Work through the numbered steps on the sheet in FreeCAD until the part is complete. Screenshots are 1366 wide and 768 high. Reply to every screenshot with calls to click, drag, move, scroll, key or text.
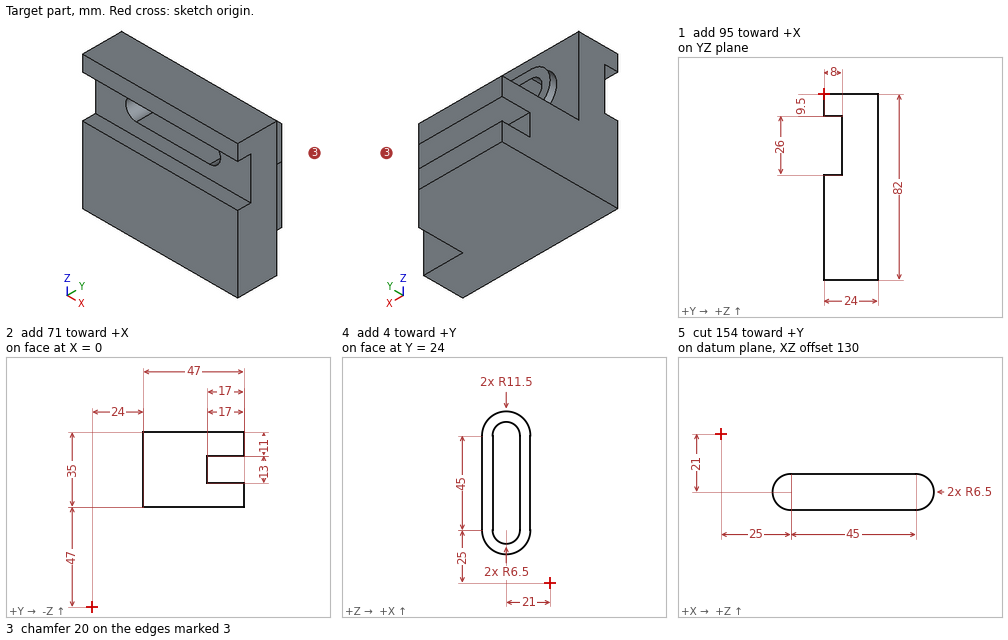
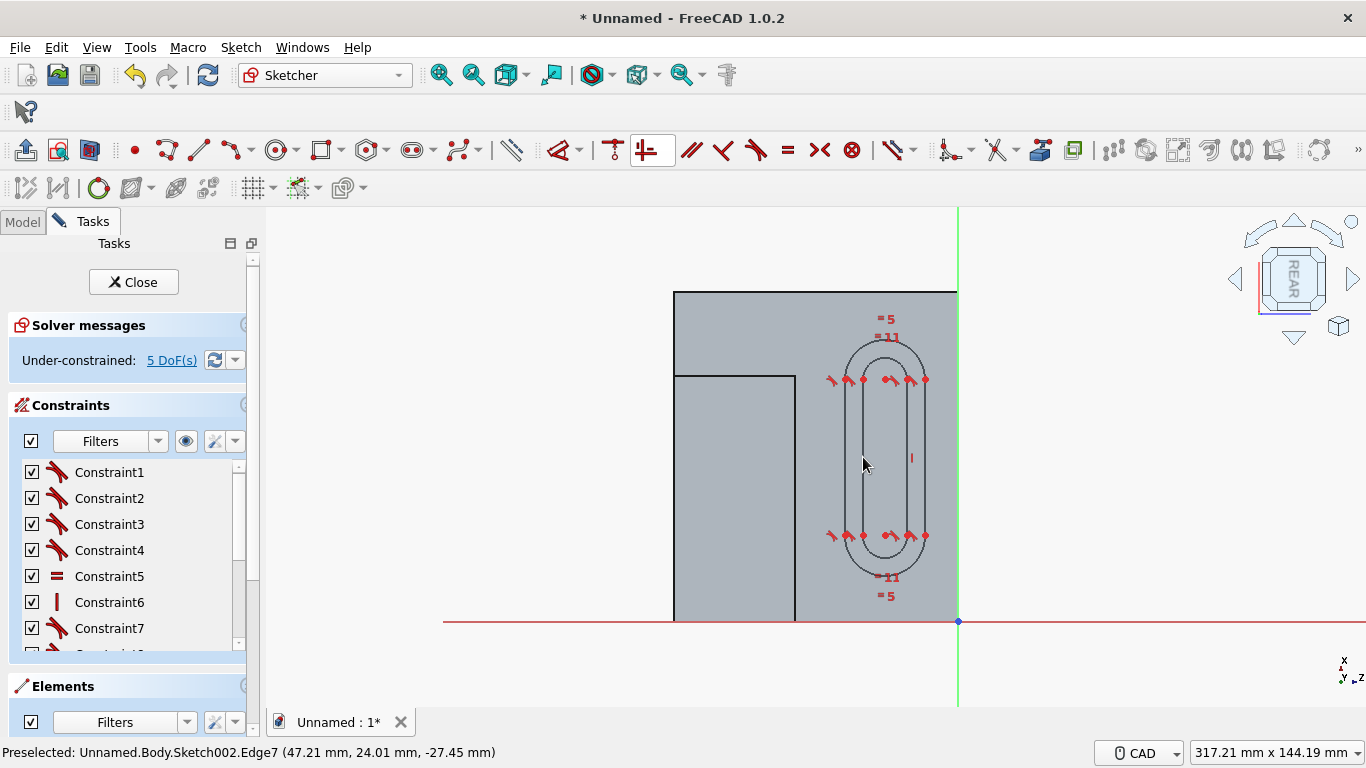
click(558, 150)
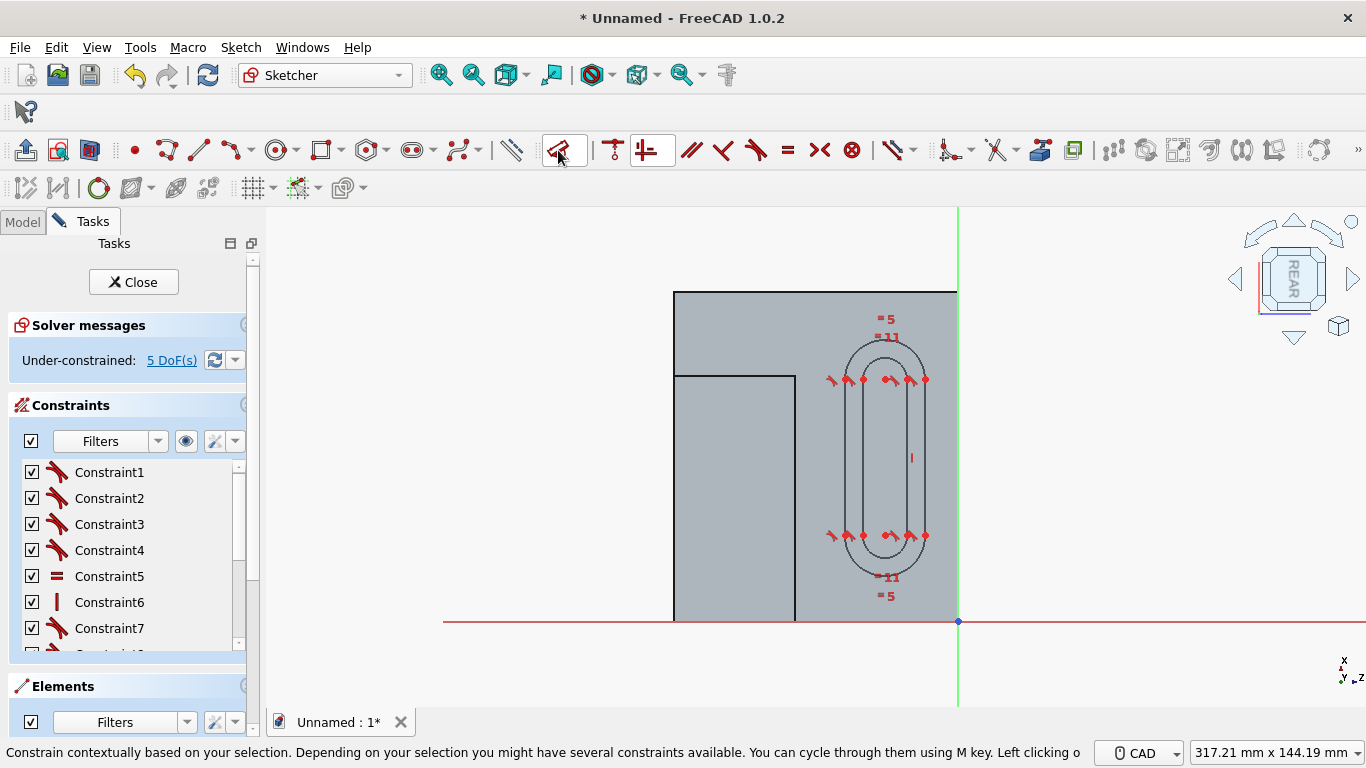
click(861, 568)
click(842, 594)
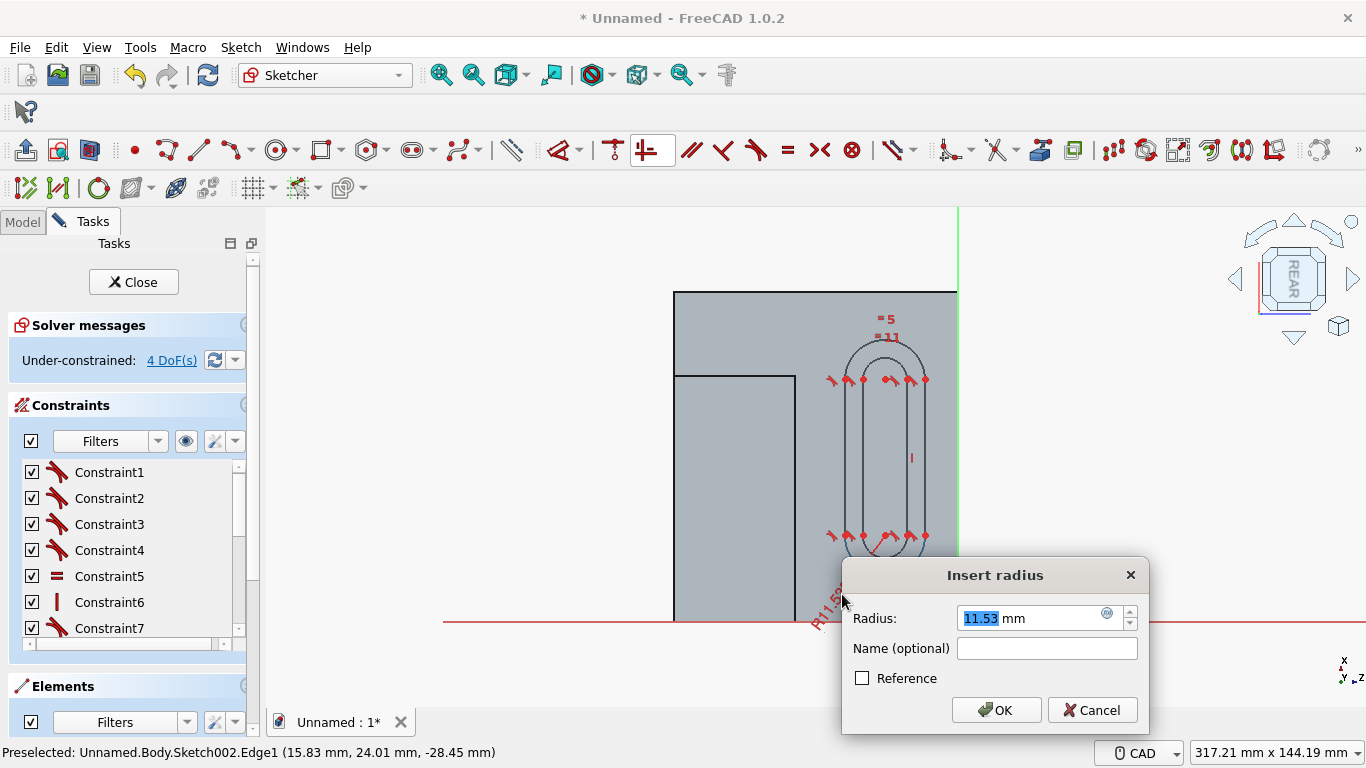
text(11.5)
key(Return)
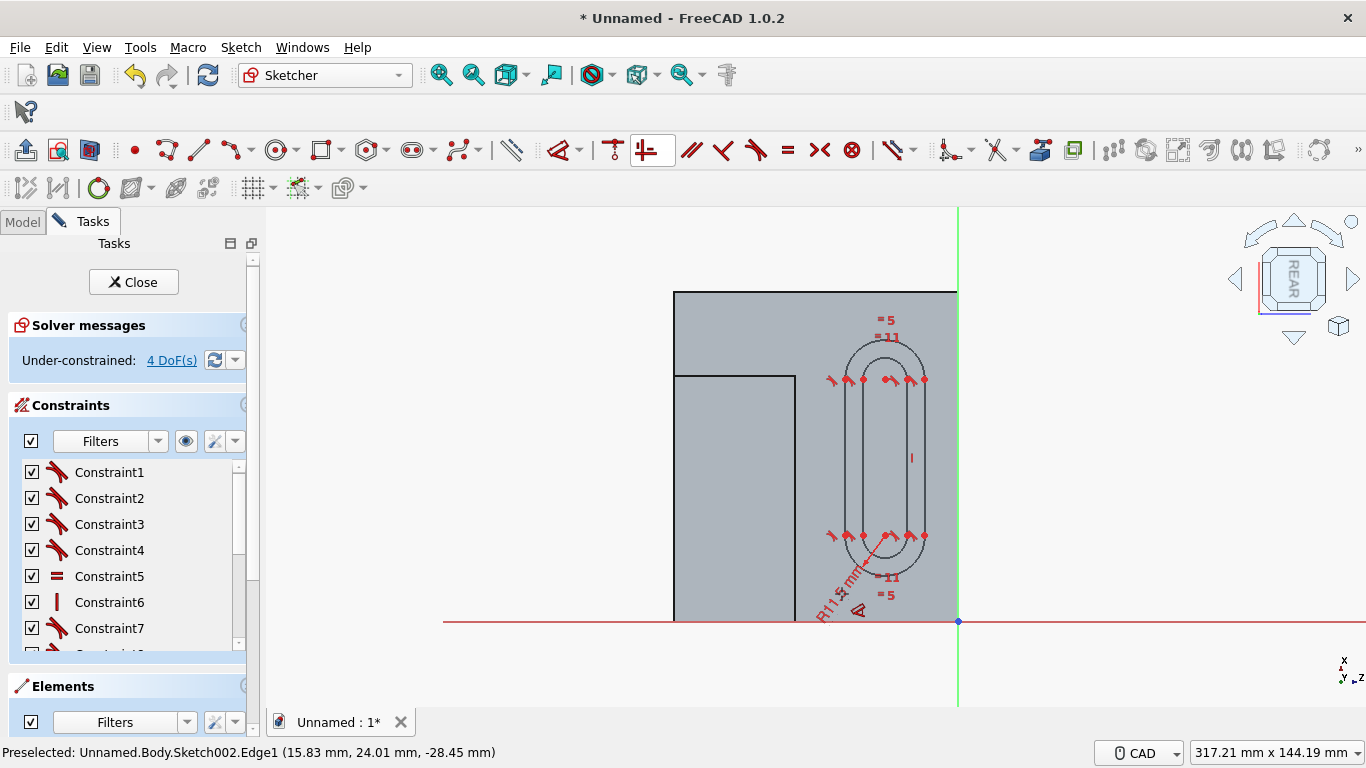
scroll(872, 554, up, 3)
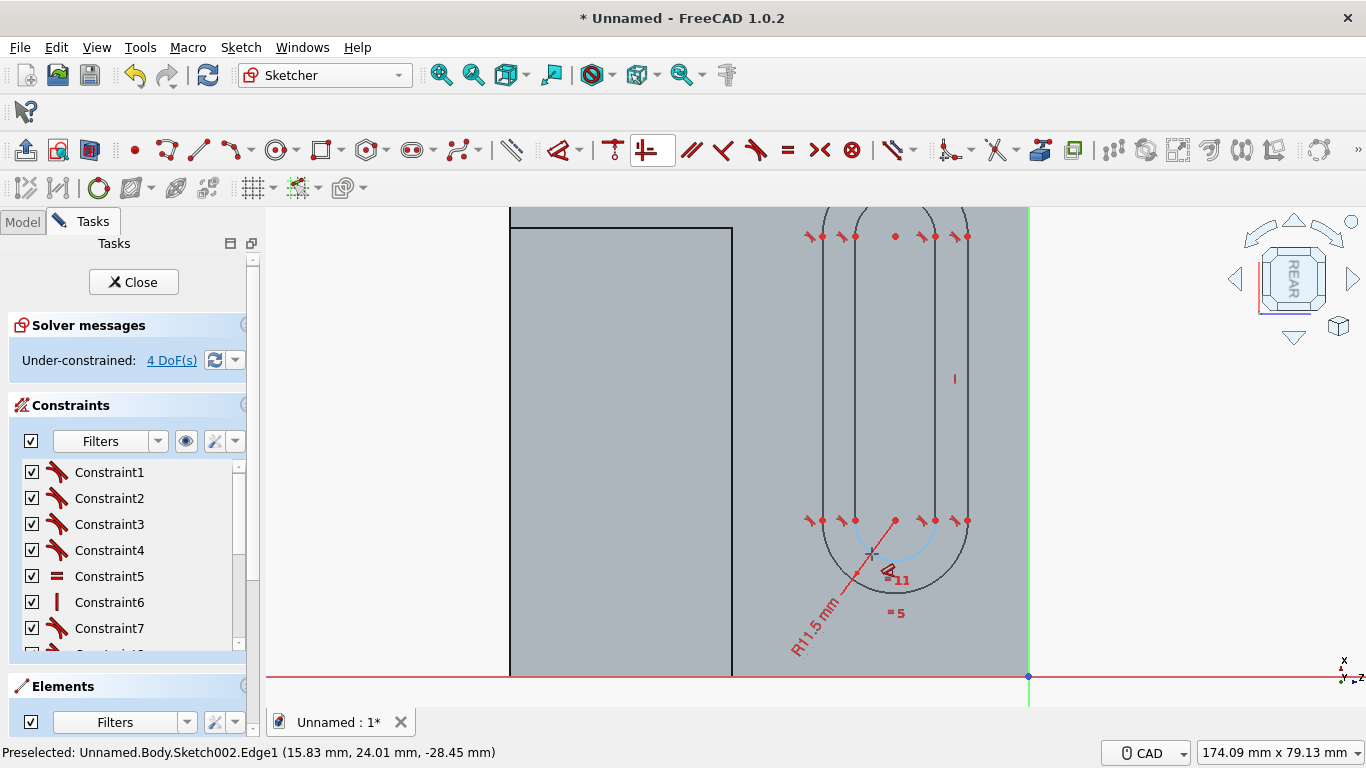
click(872, 553)
click(837, 479)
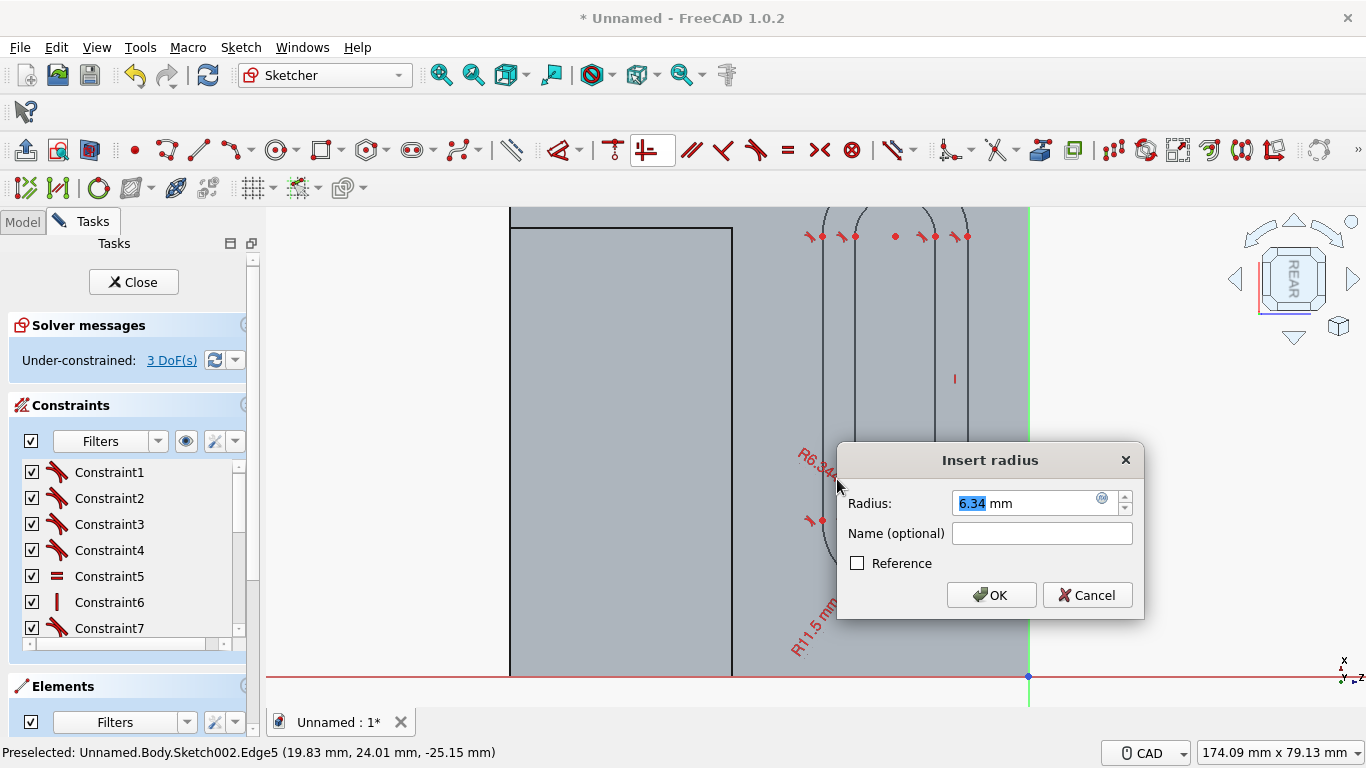
text(6.5)
key(Return)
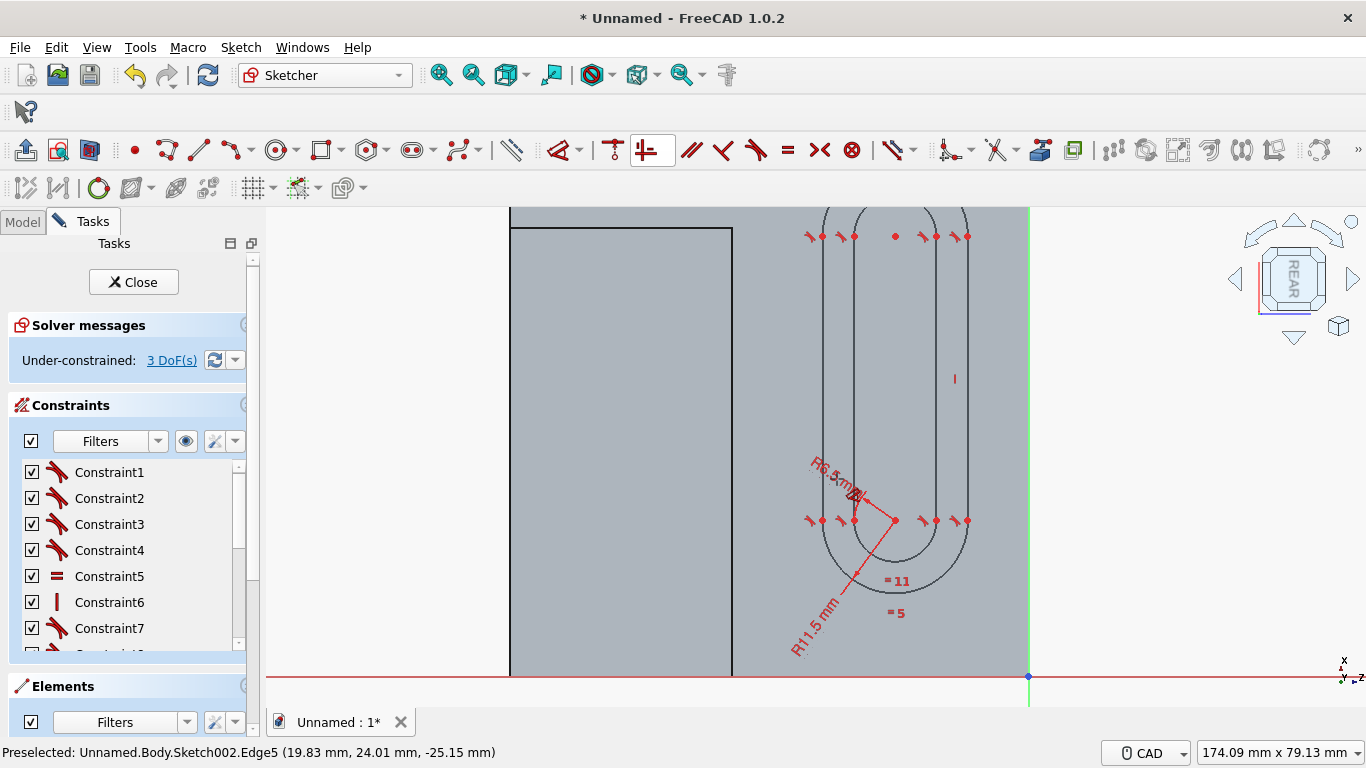
click(823, 435)
click(789, 379)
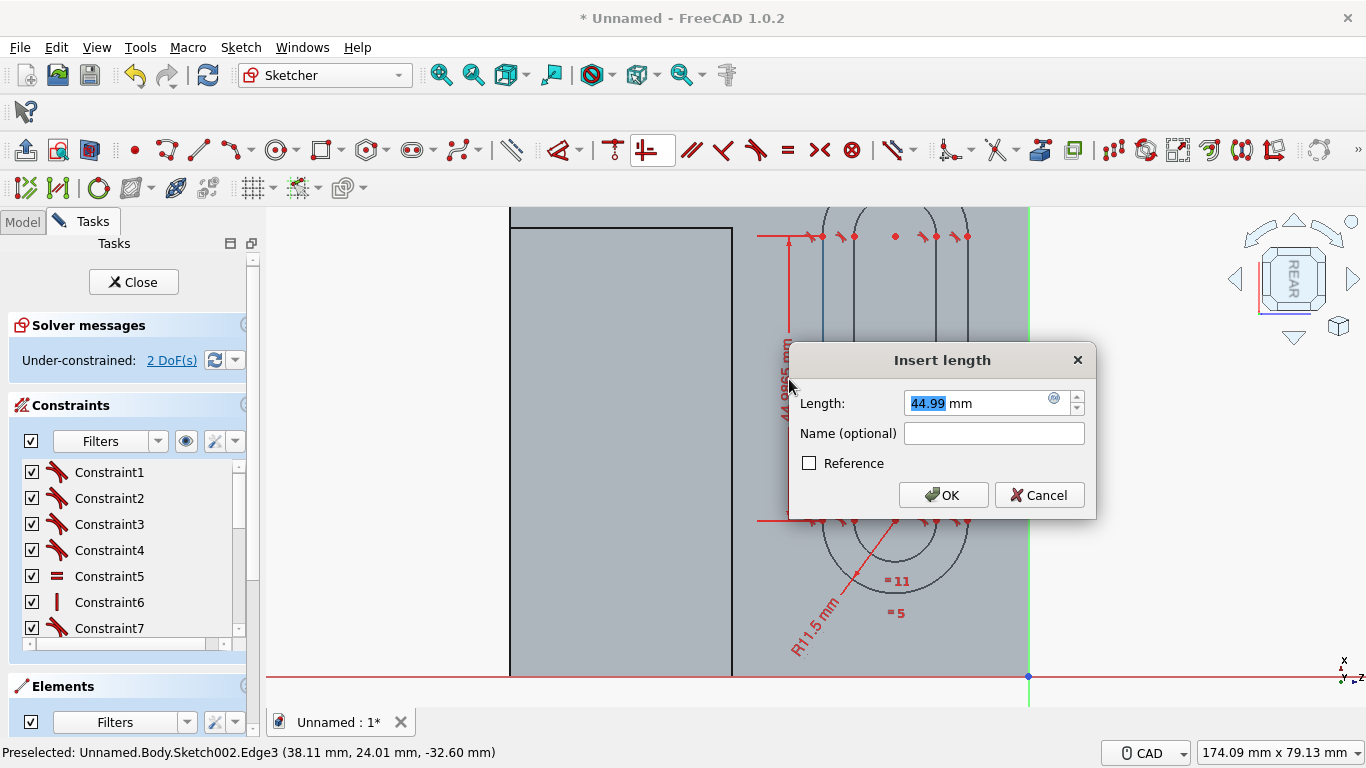
text(45)
key(Return)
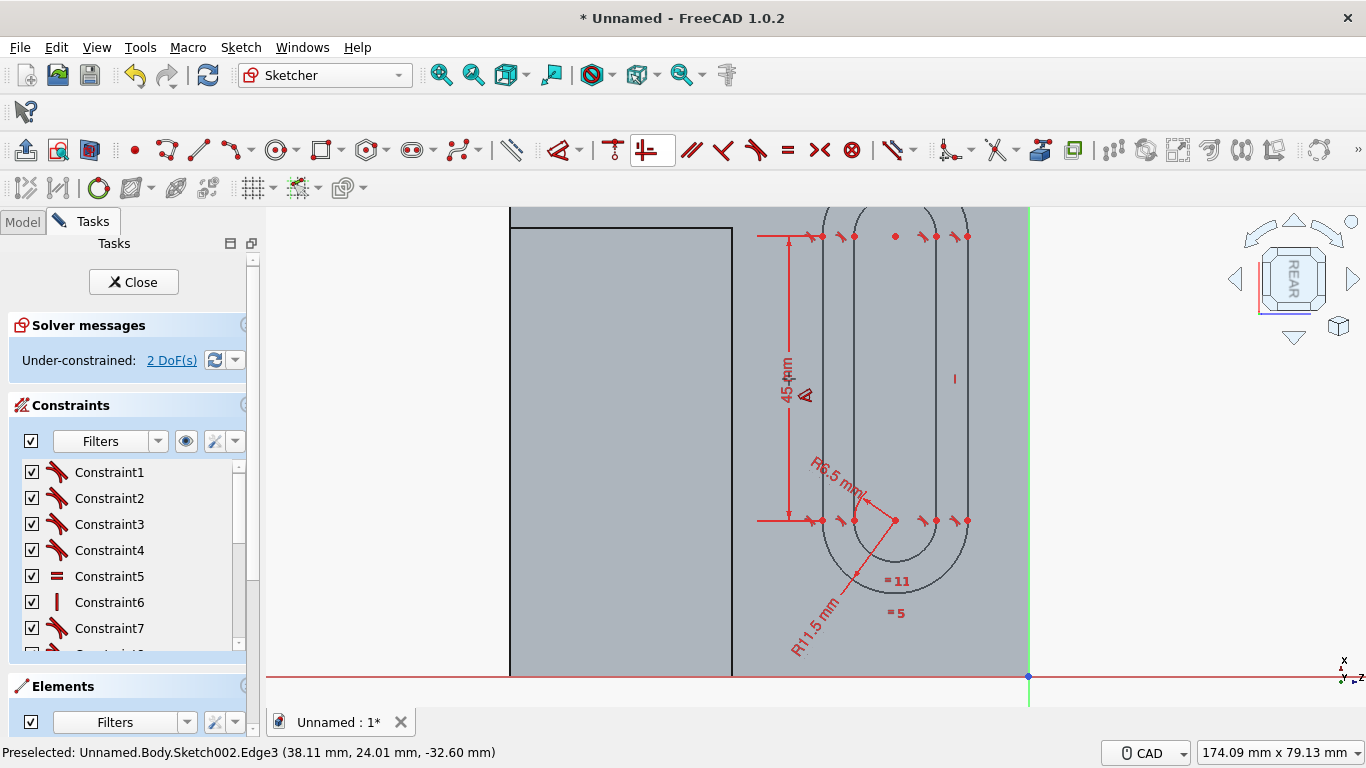
click(823, 521)
click(789, 599)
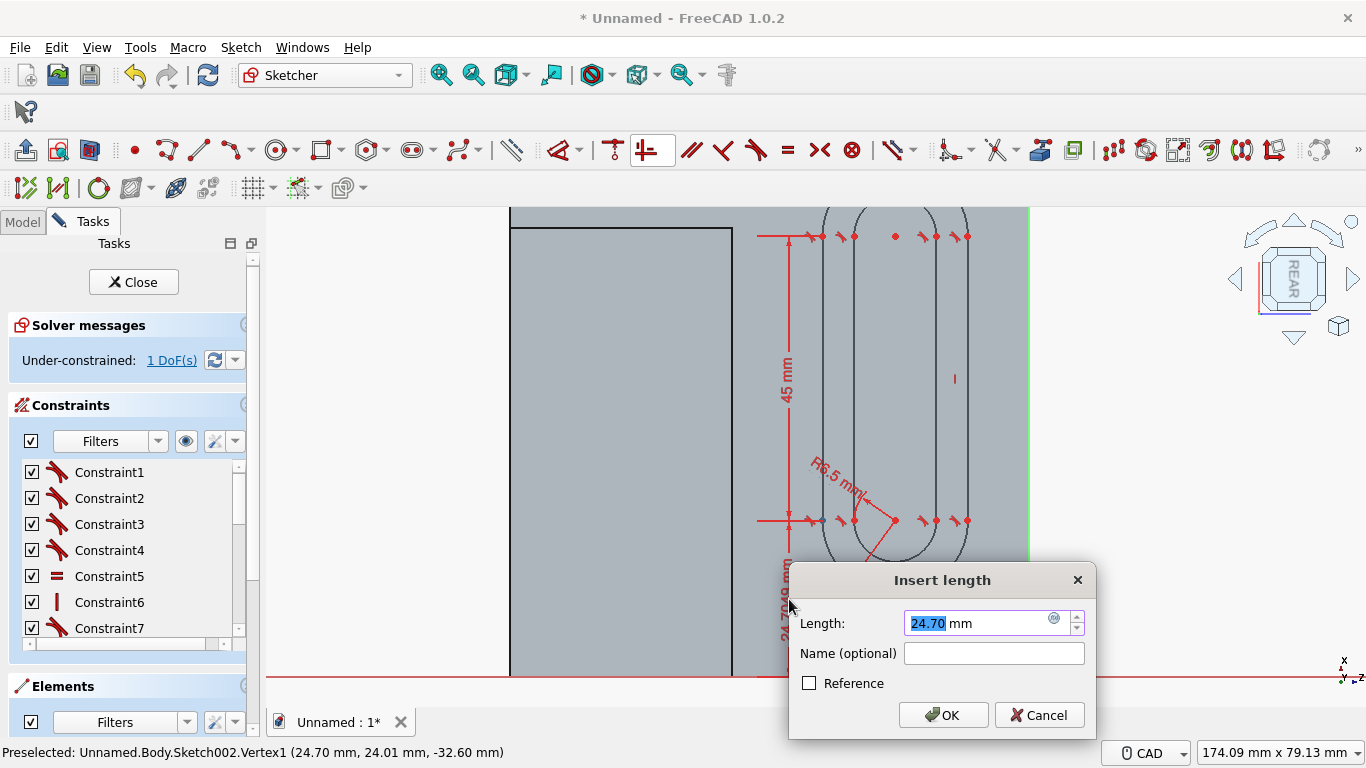
text(25)
key(Return)